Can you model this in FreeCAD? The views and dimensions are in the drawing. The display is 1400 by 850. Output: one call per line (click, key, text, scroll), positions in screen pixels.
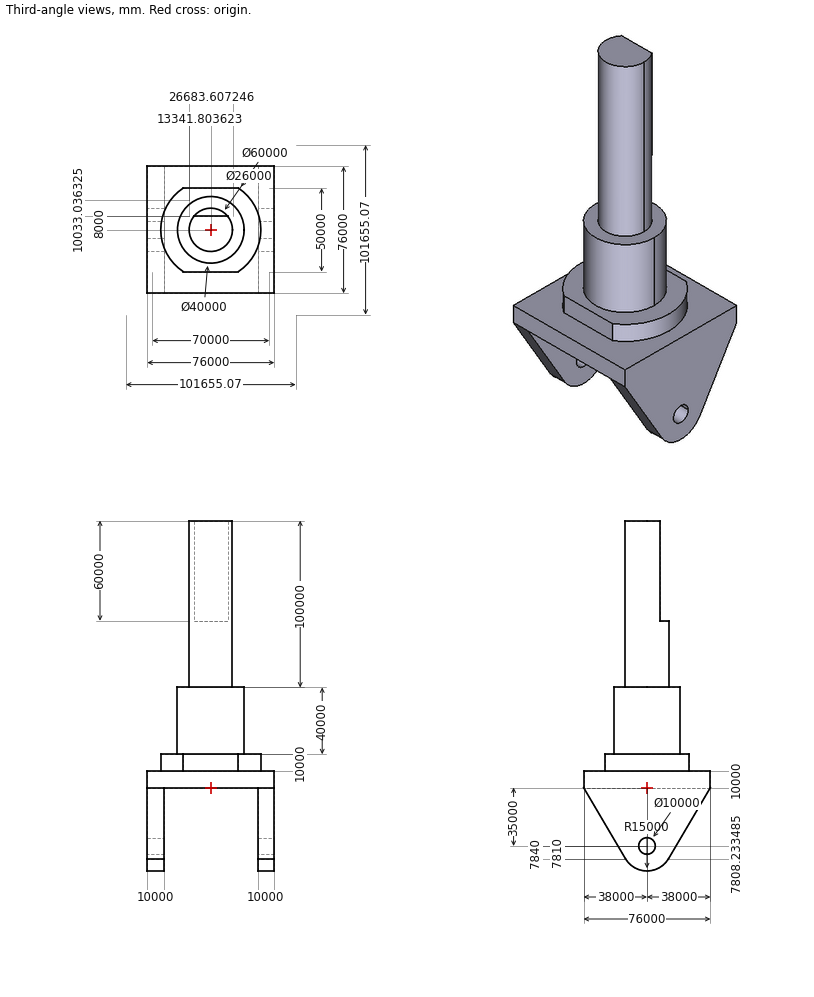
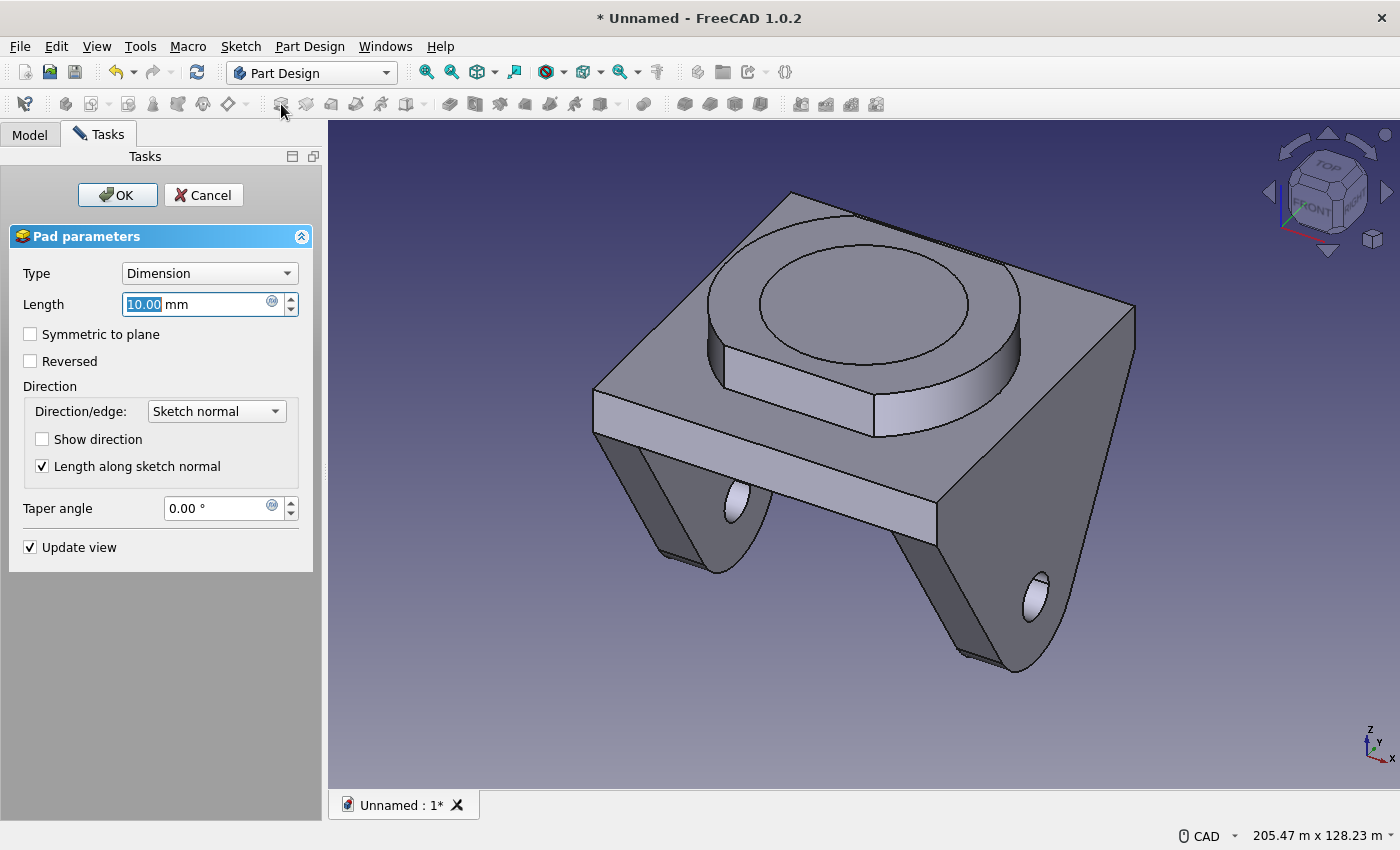
text(40000)
key(Tab)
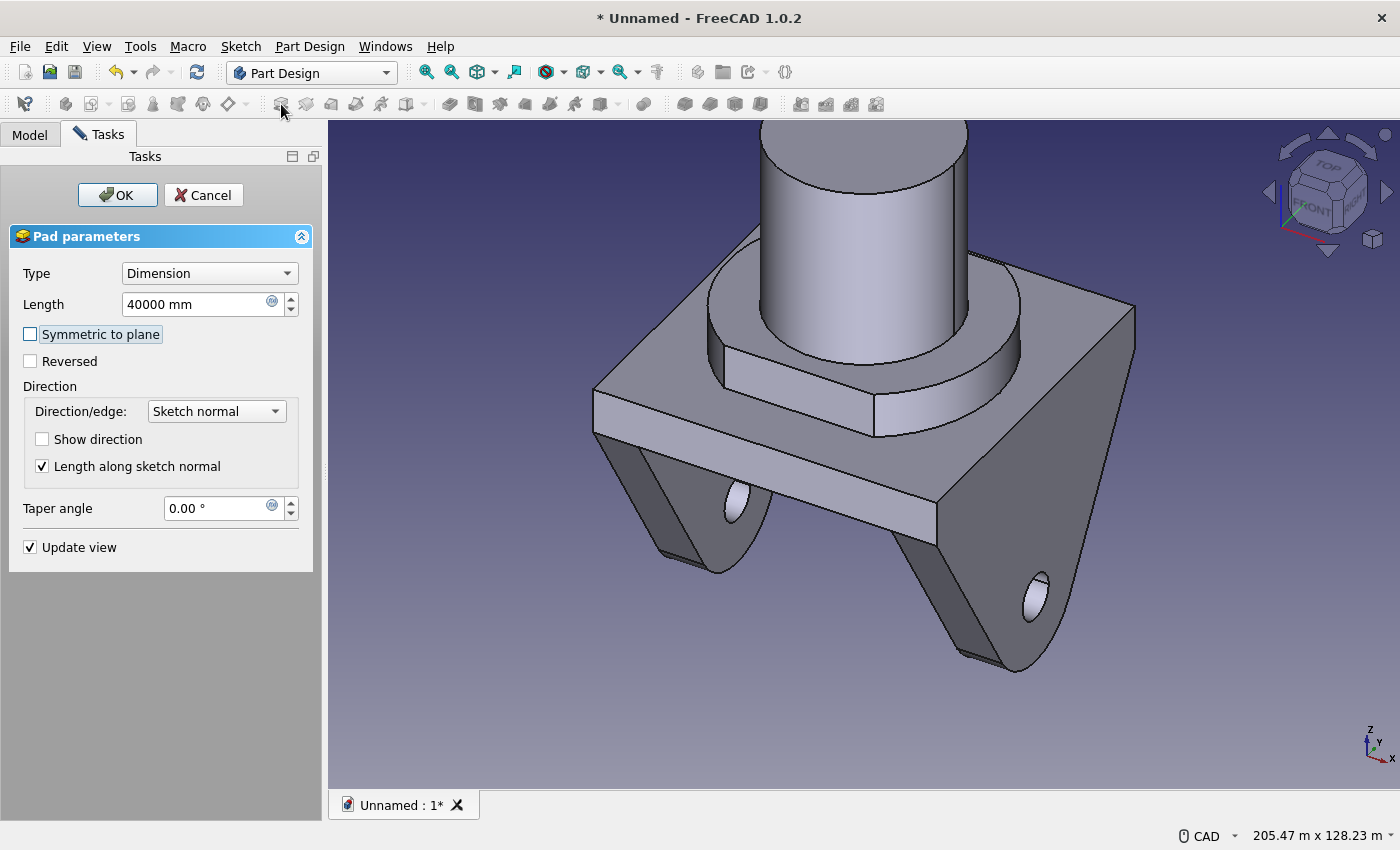
click(118, 195)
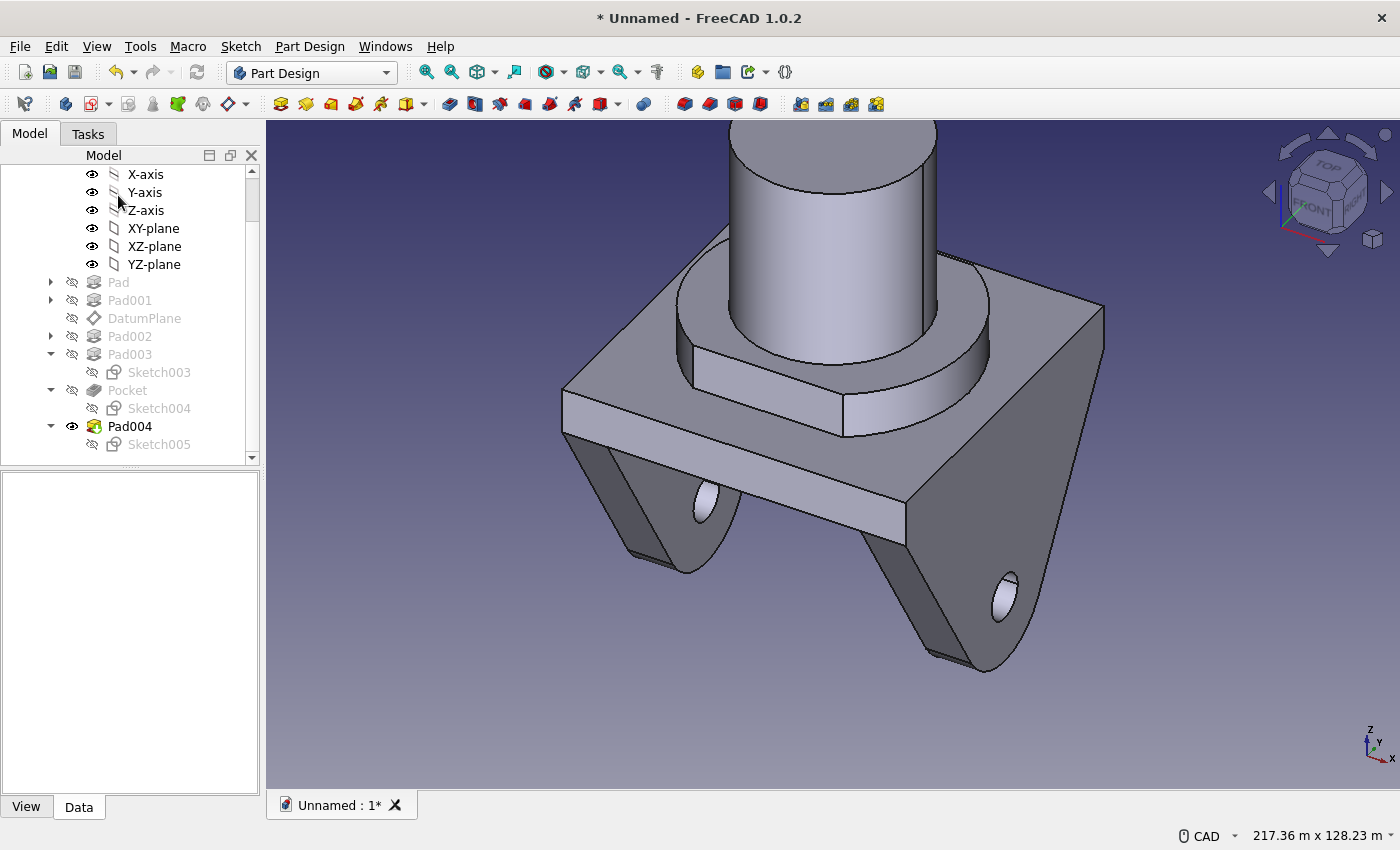
click(427, 72)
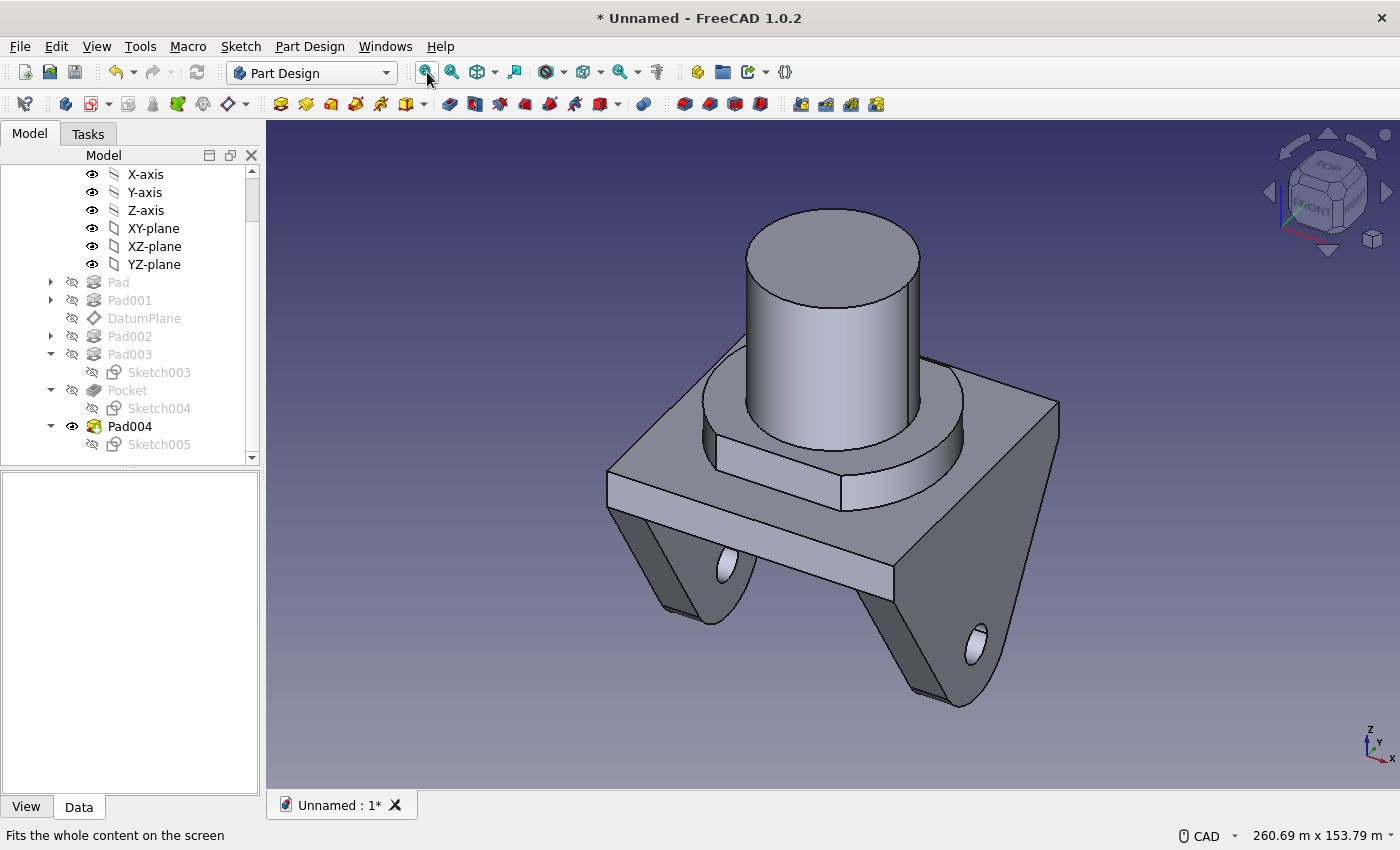
click(833, 258)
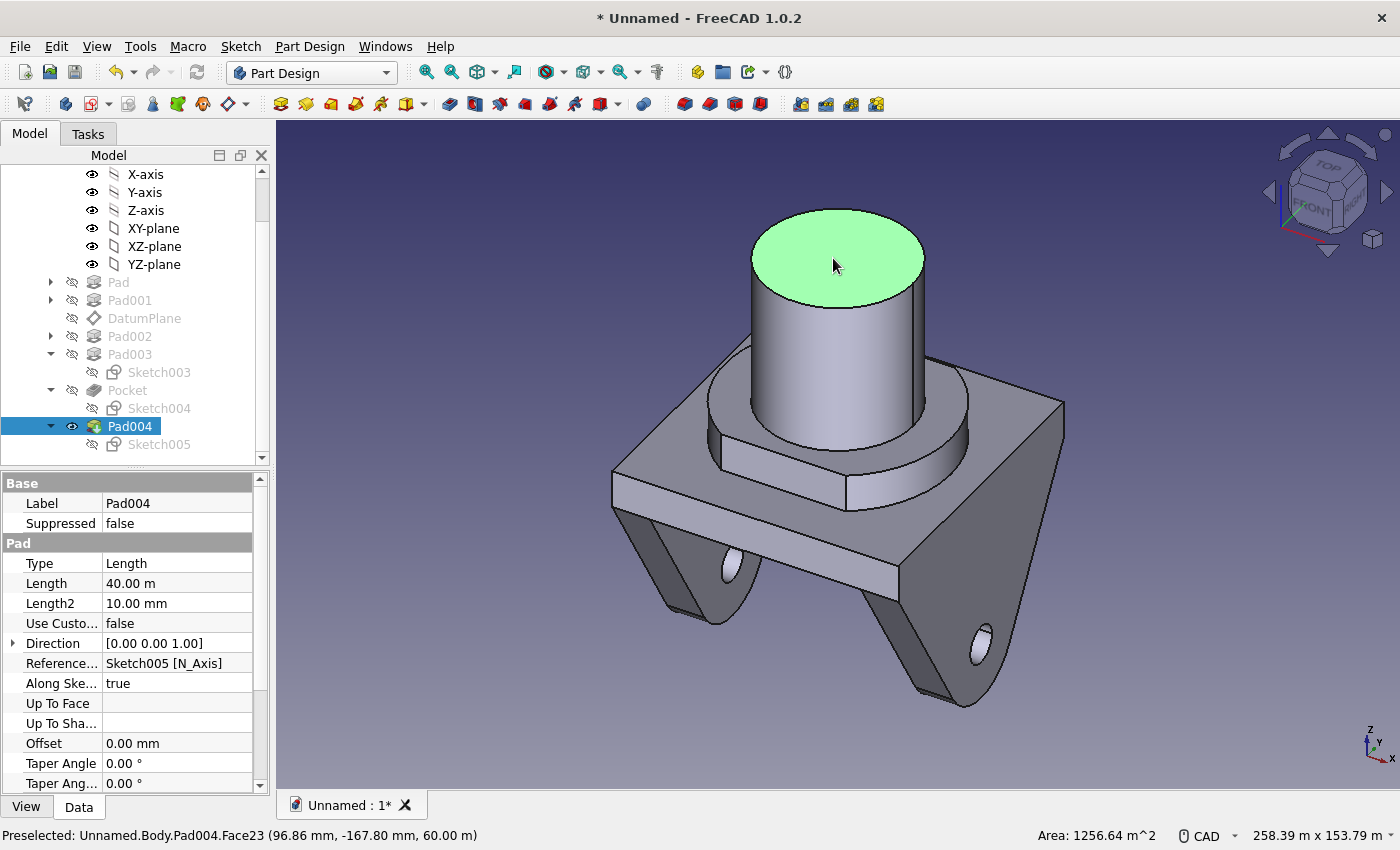
click(90, 104)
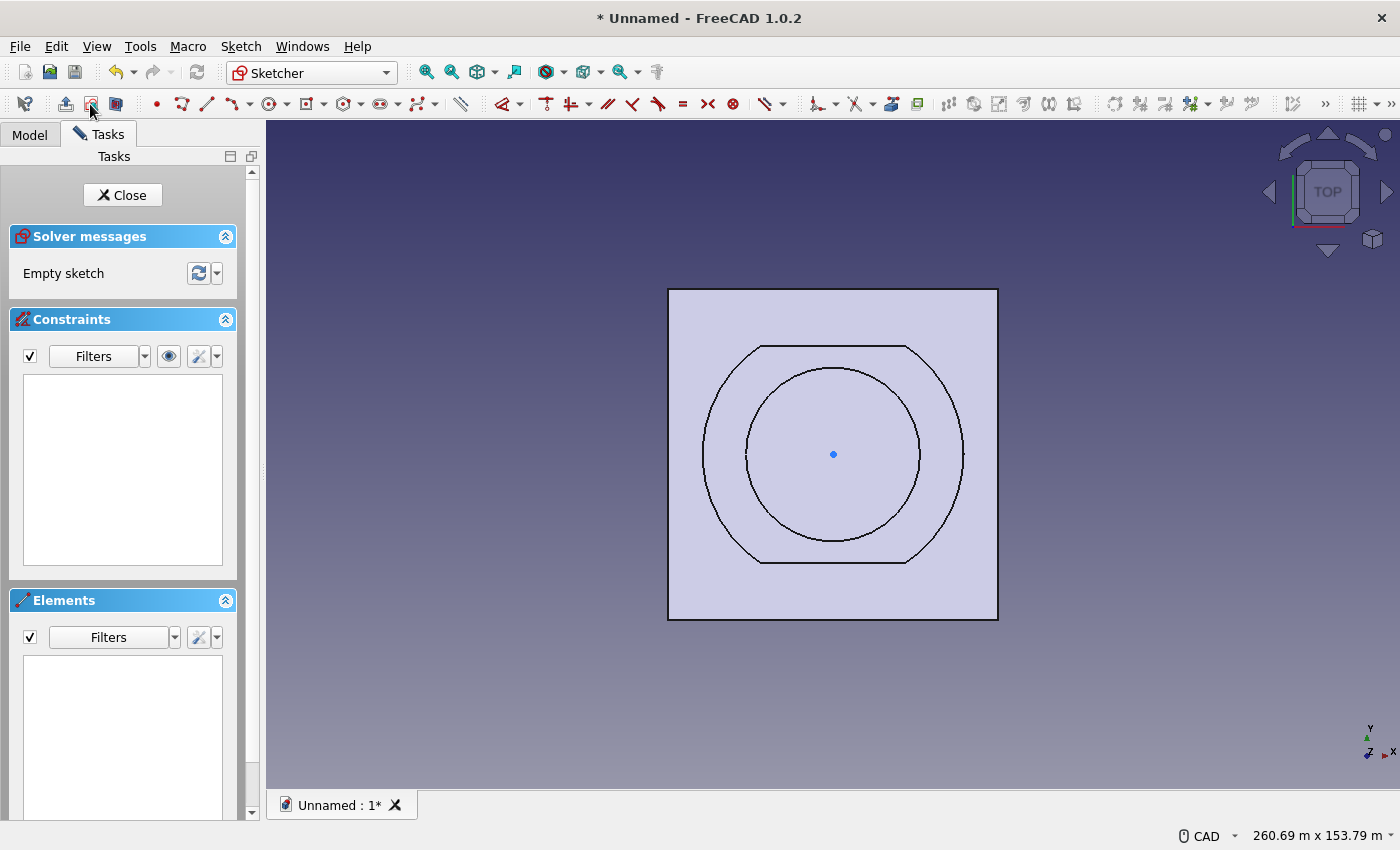
scroll(855, 454, up, 7)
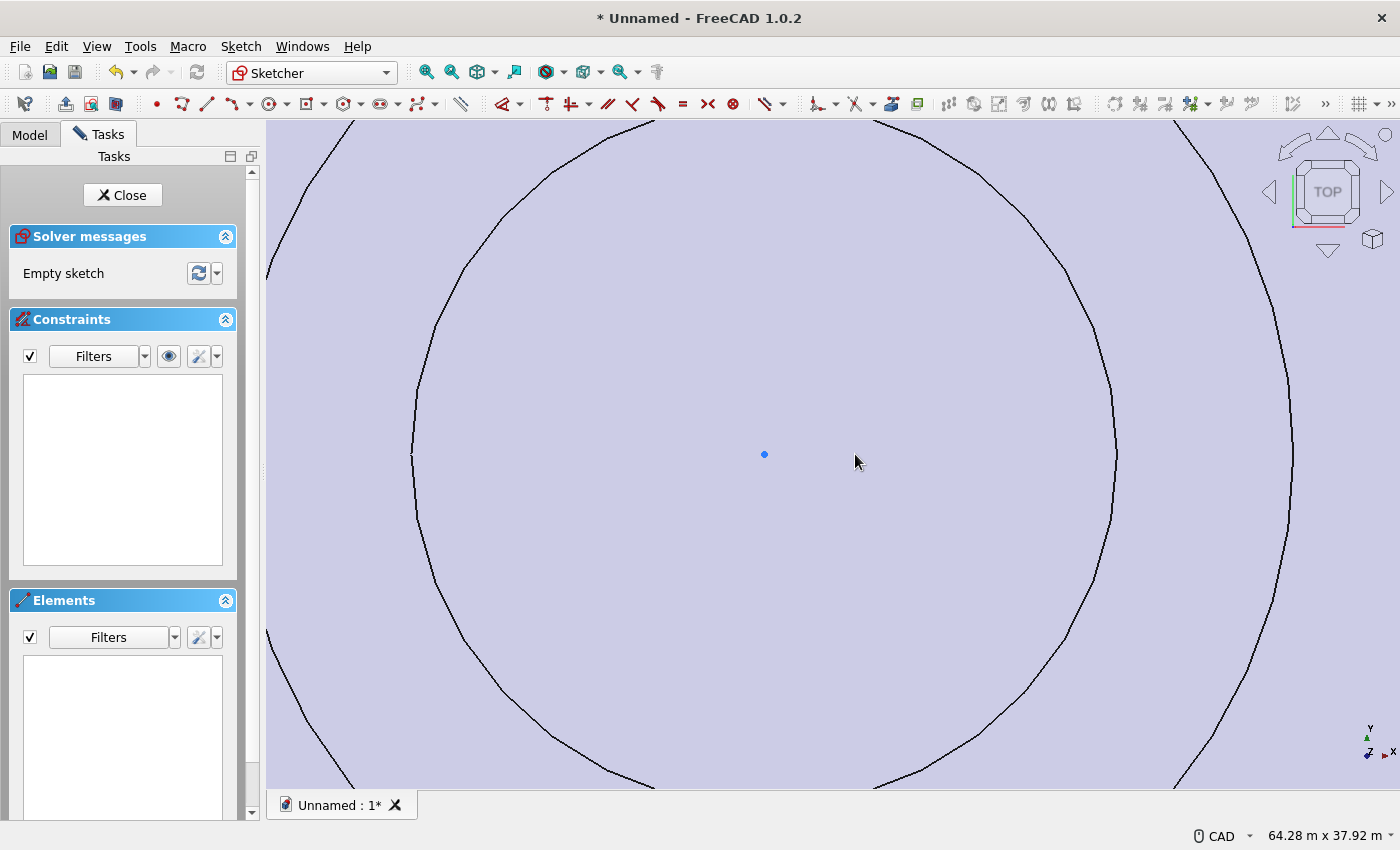
click(268, 104)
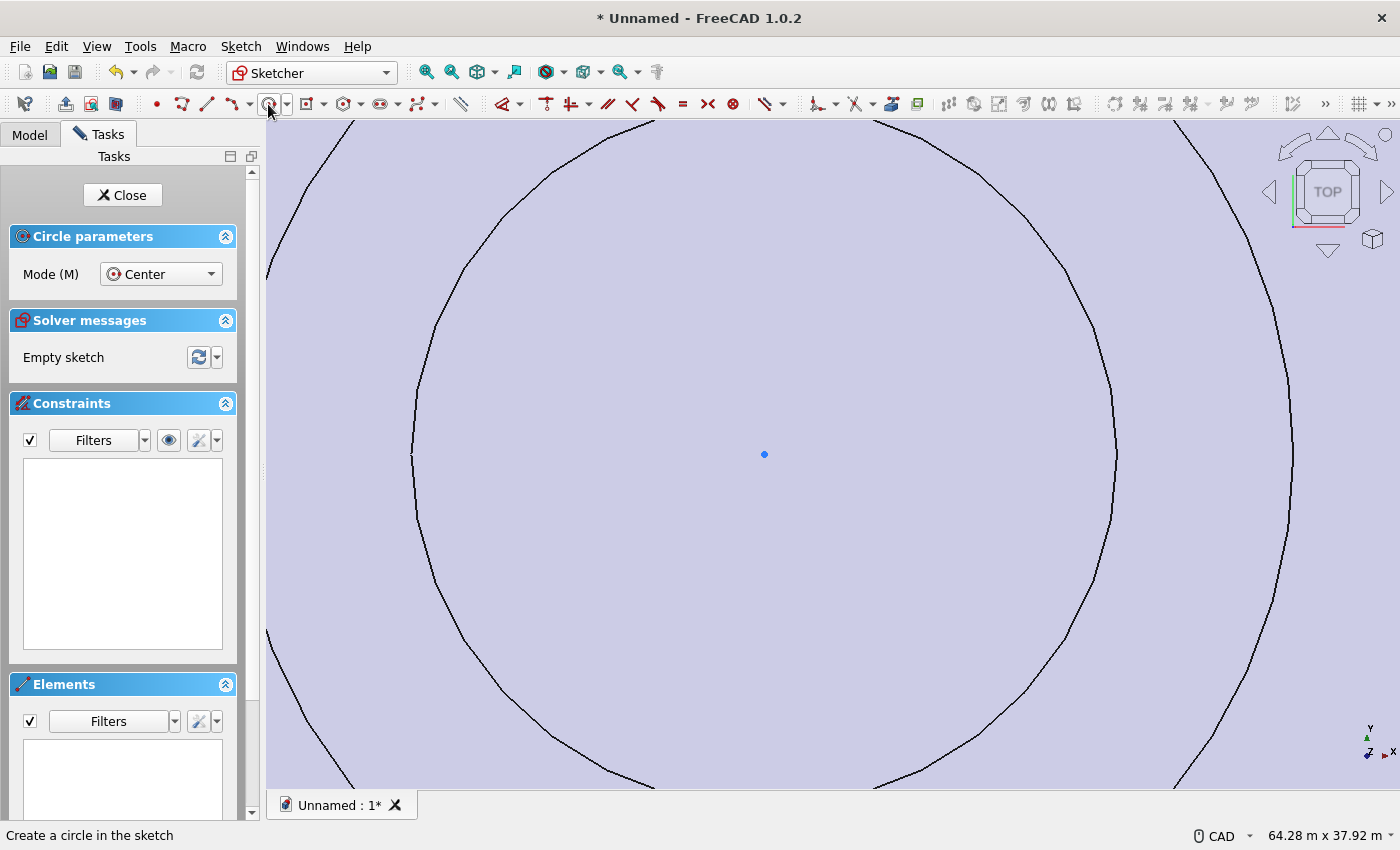
click(764, 454)
click(926, 292)
key(Escape)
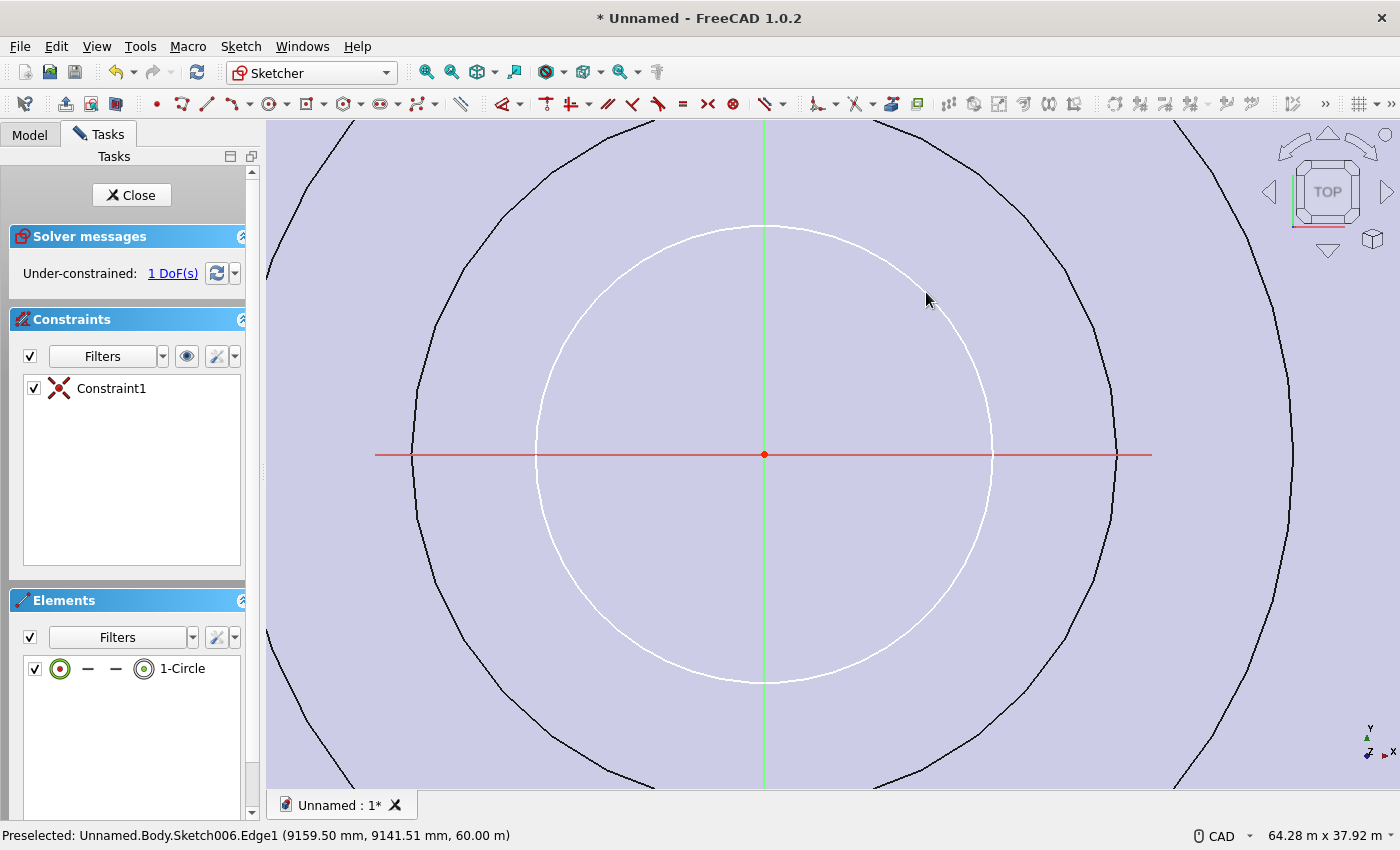
click(502, 104)